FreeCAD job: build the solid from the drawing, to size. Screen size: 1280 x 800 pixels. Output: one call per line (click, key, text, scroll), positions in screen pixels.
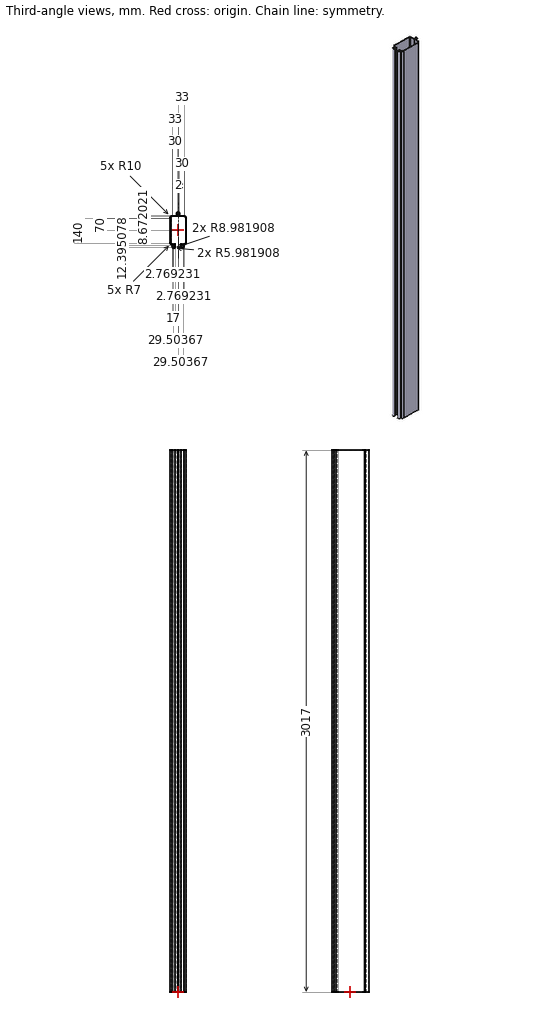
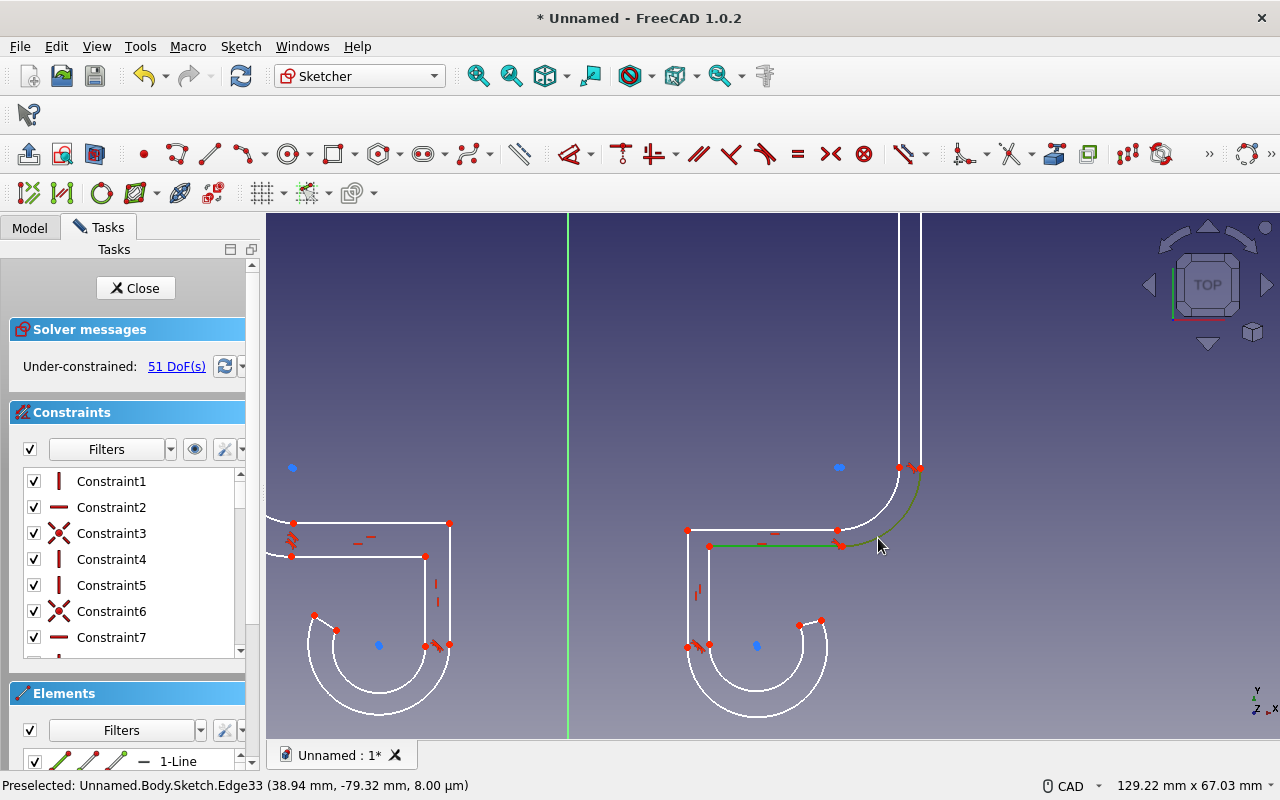
click(765, 154)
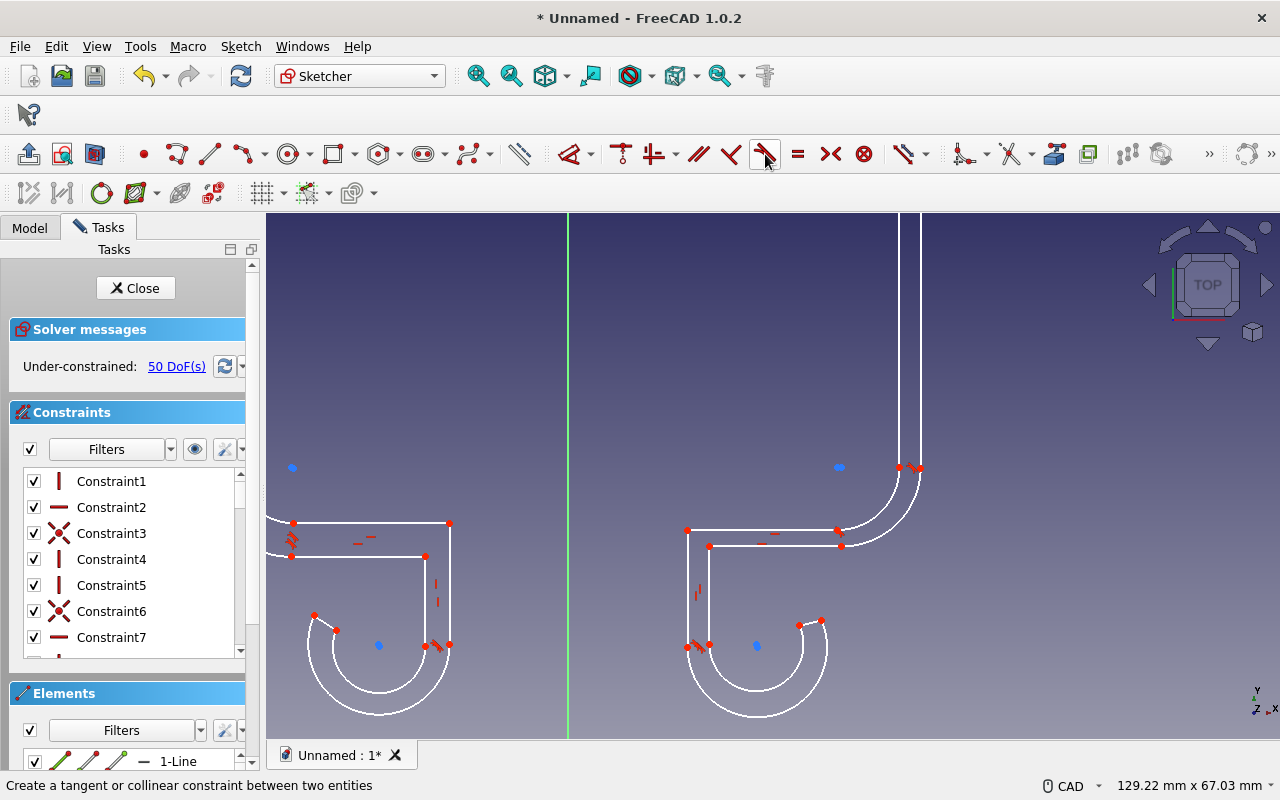
click(921, 249)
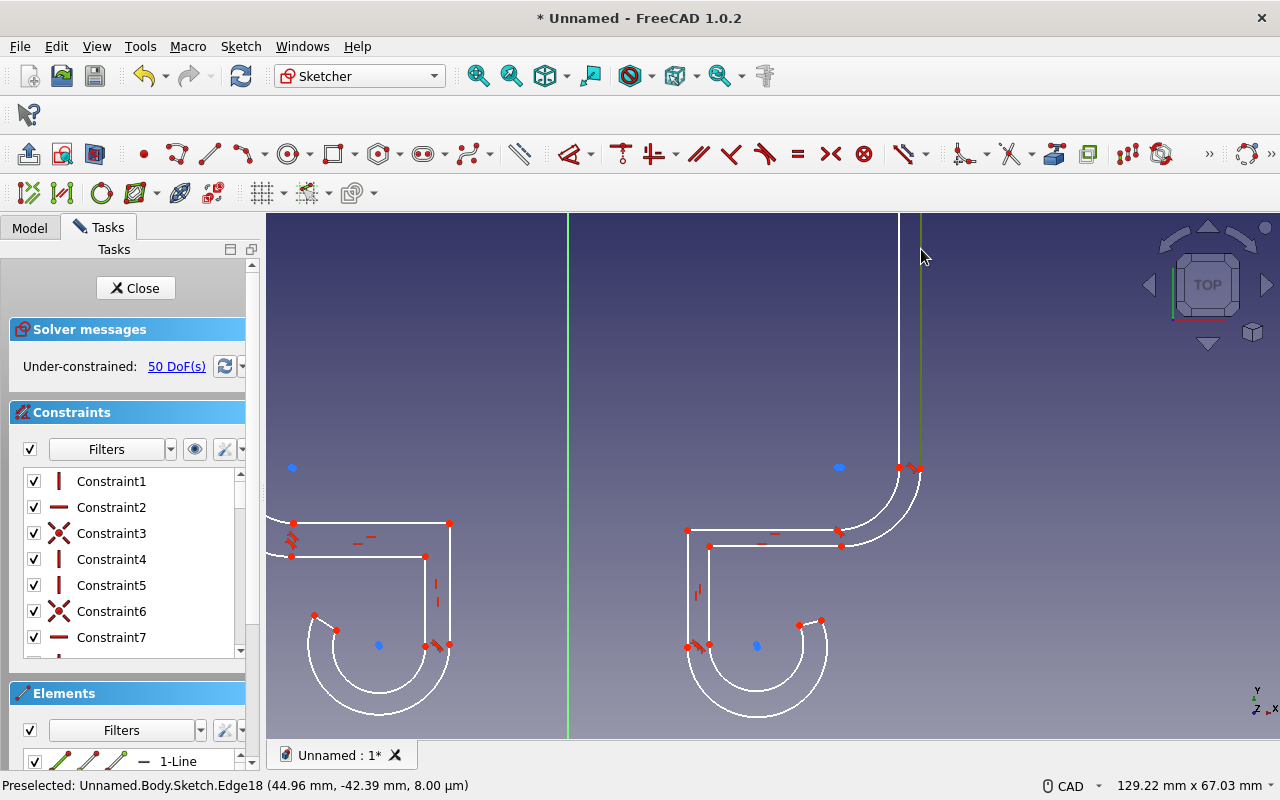
click(877, 538)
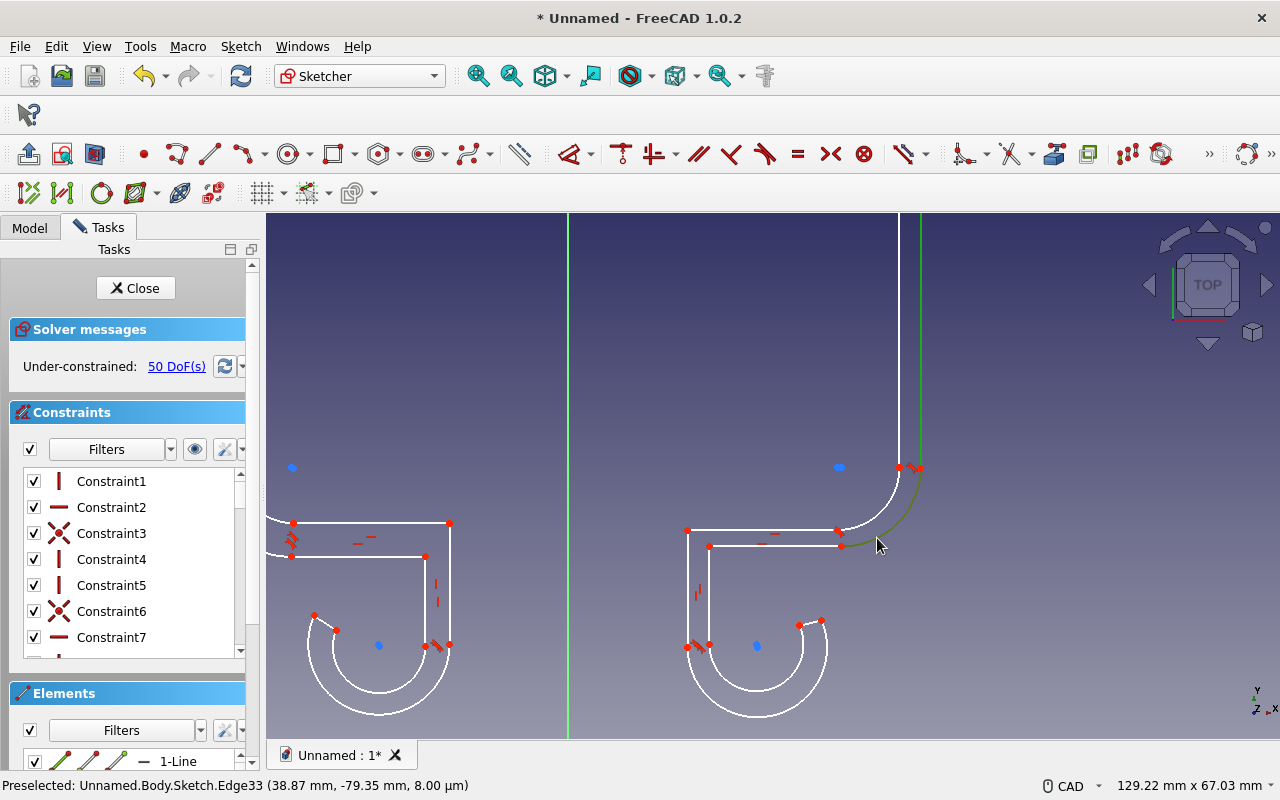
click(765, 154)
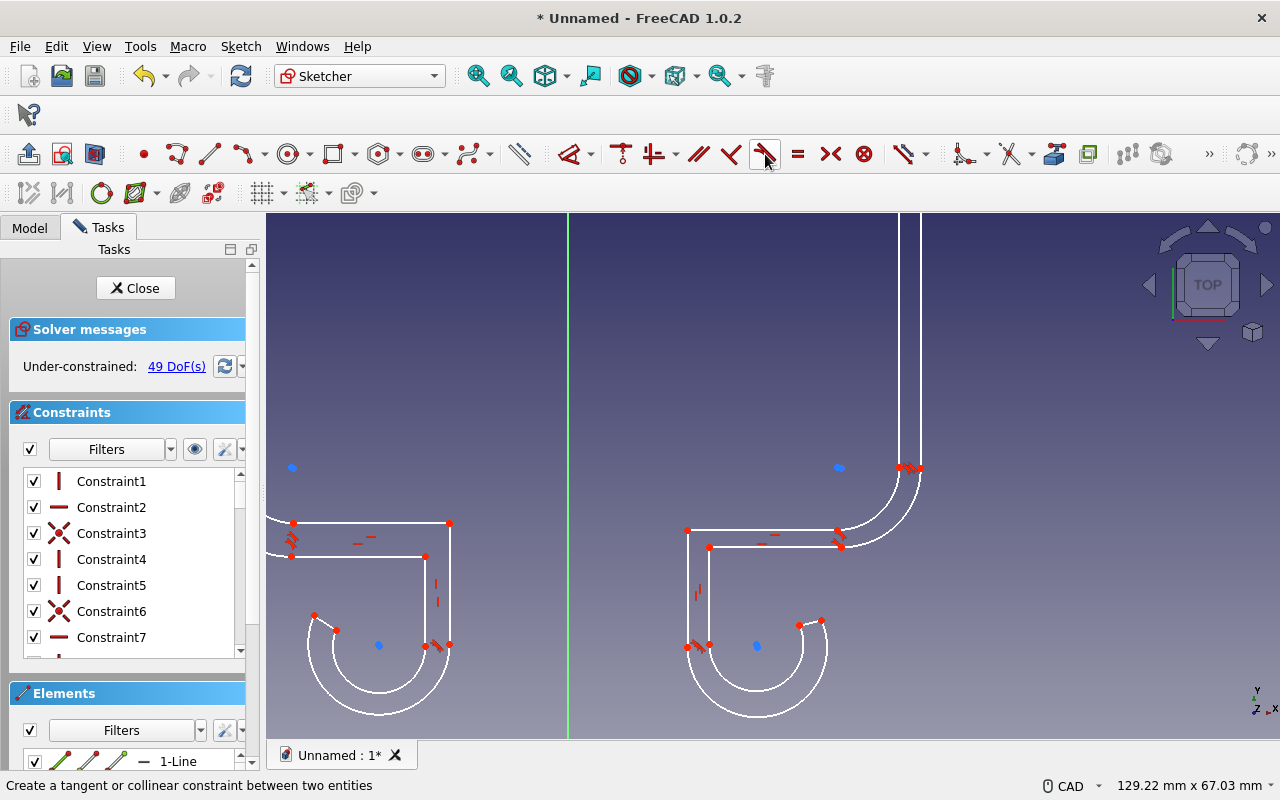
click(921, 249)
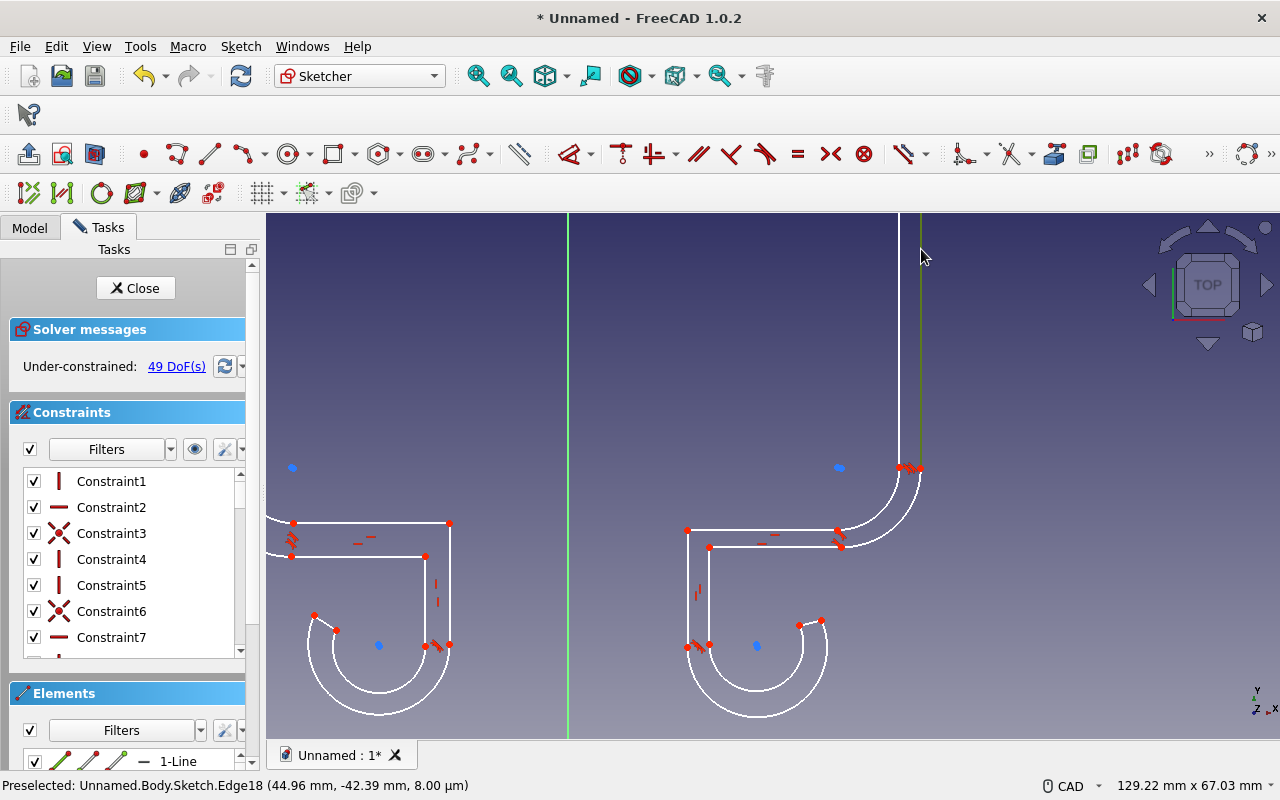
scroll(739, 618, down, 8)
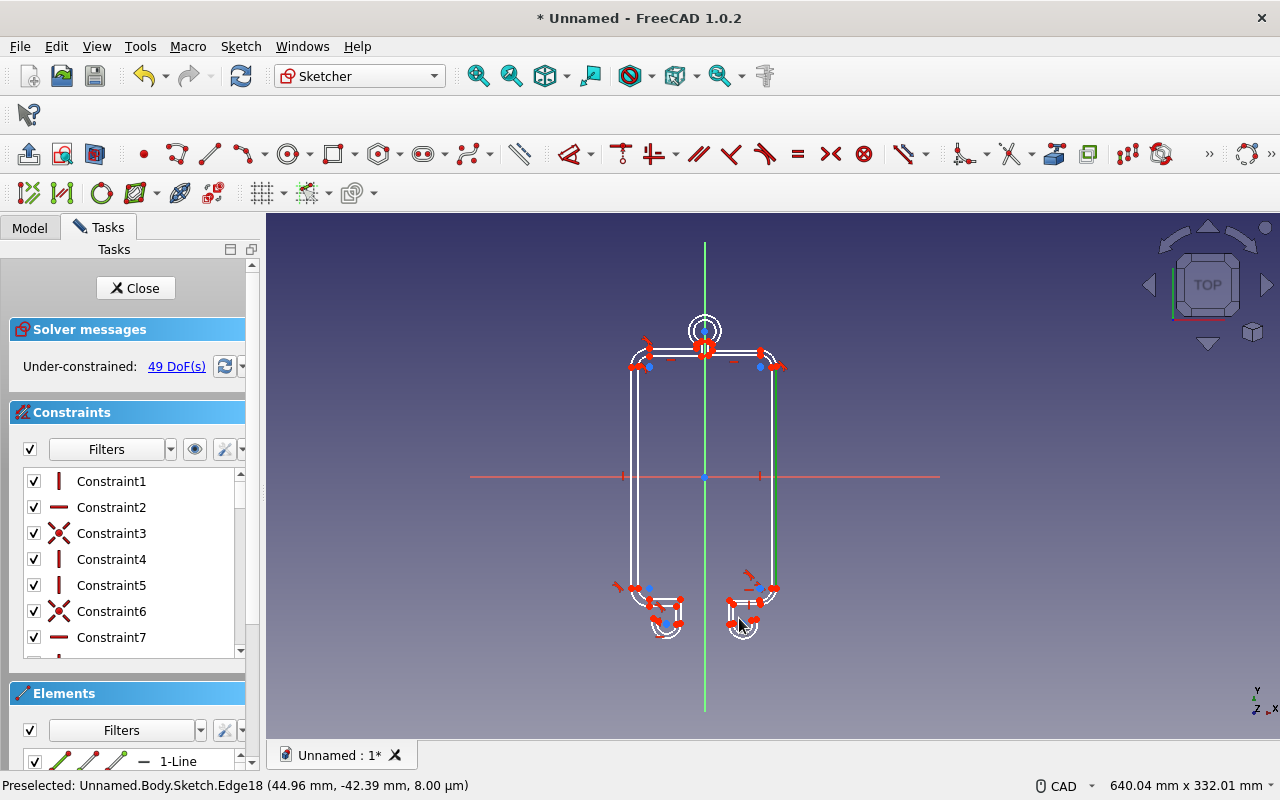
scroll(774, 359, up, 6)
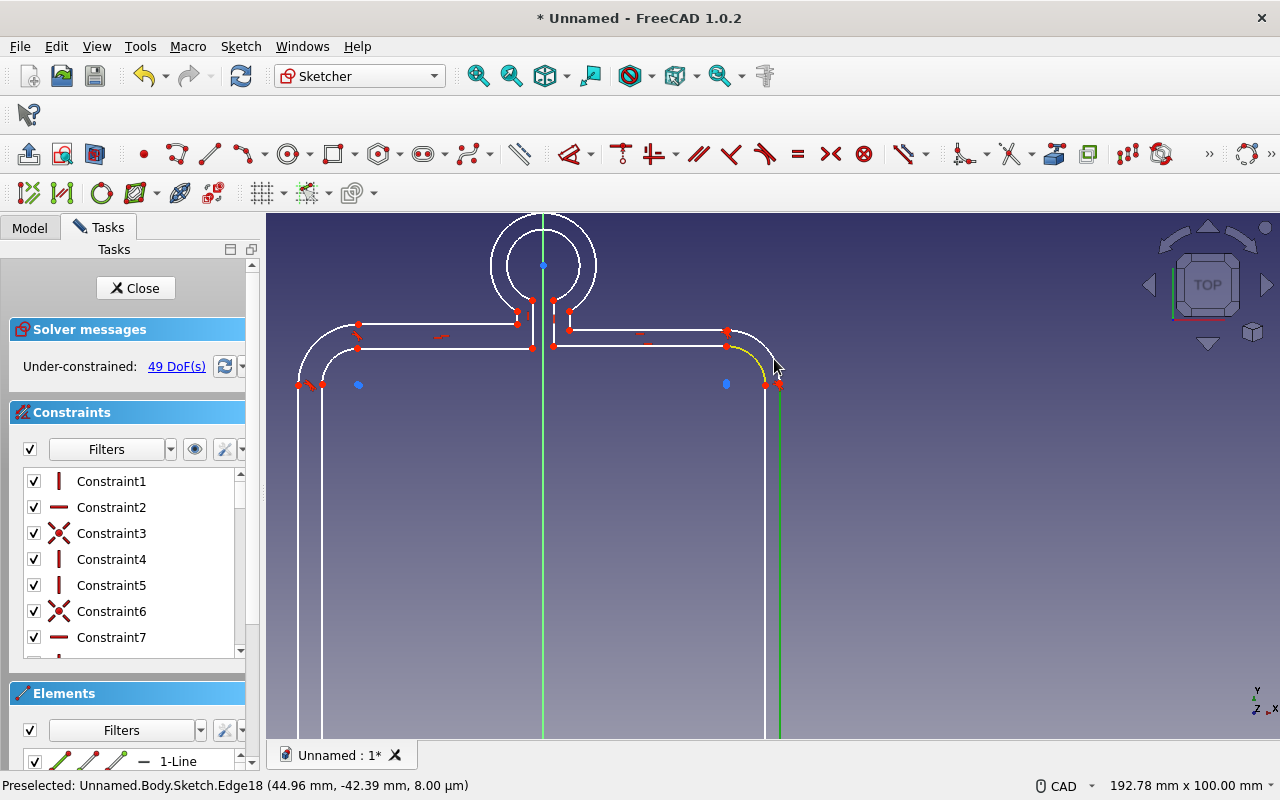
click(774, 360)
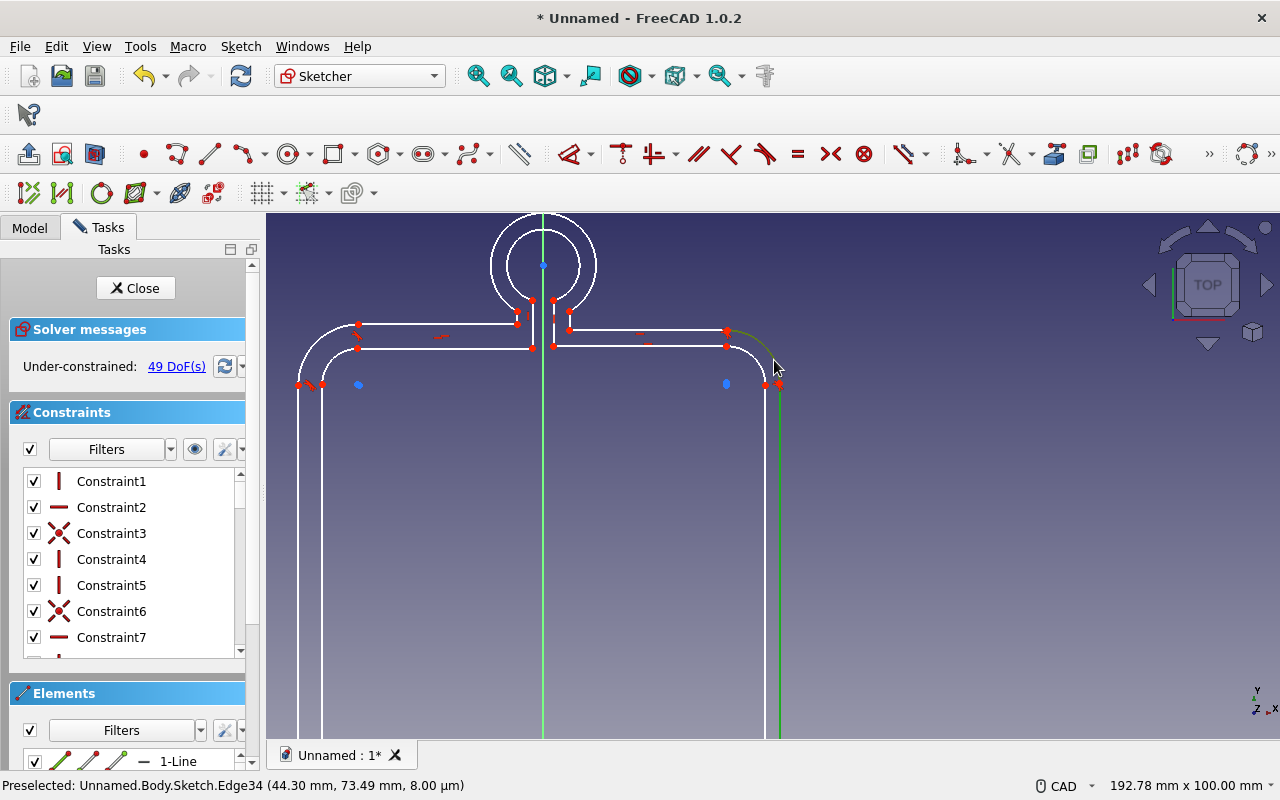
click(765, 154)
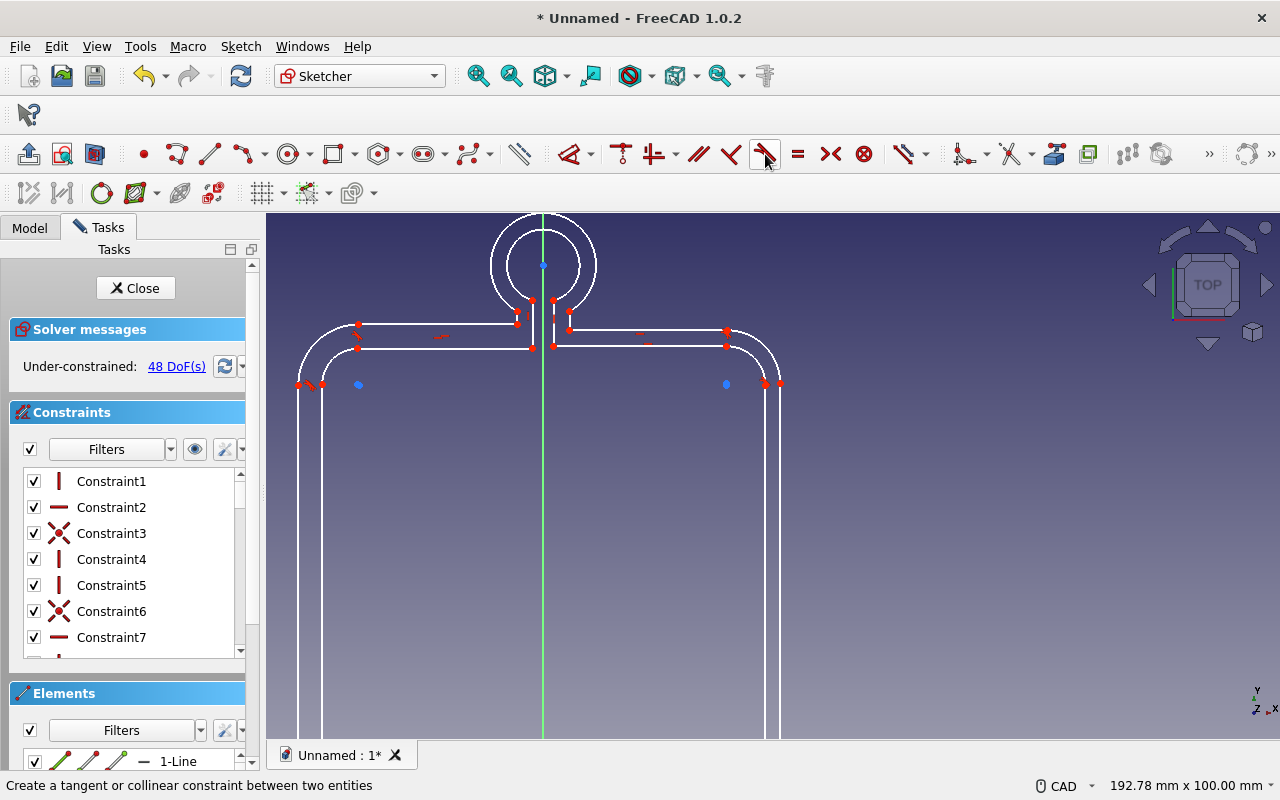
click(680, 330)